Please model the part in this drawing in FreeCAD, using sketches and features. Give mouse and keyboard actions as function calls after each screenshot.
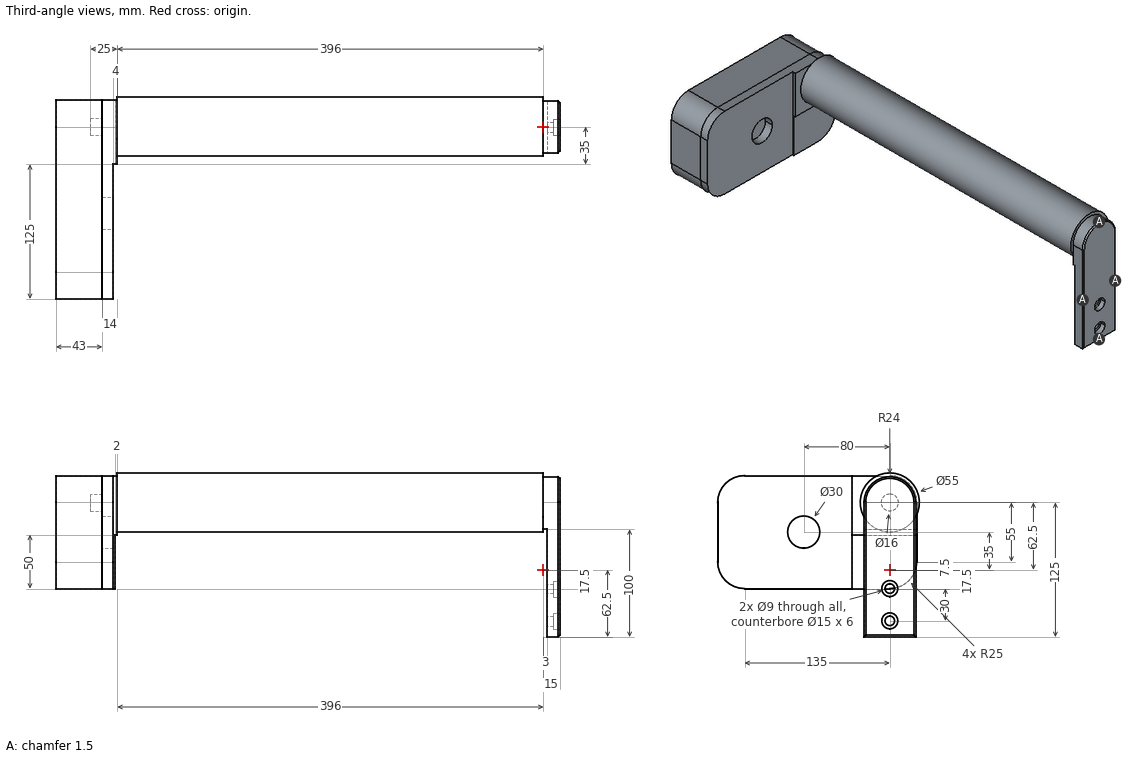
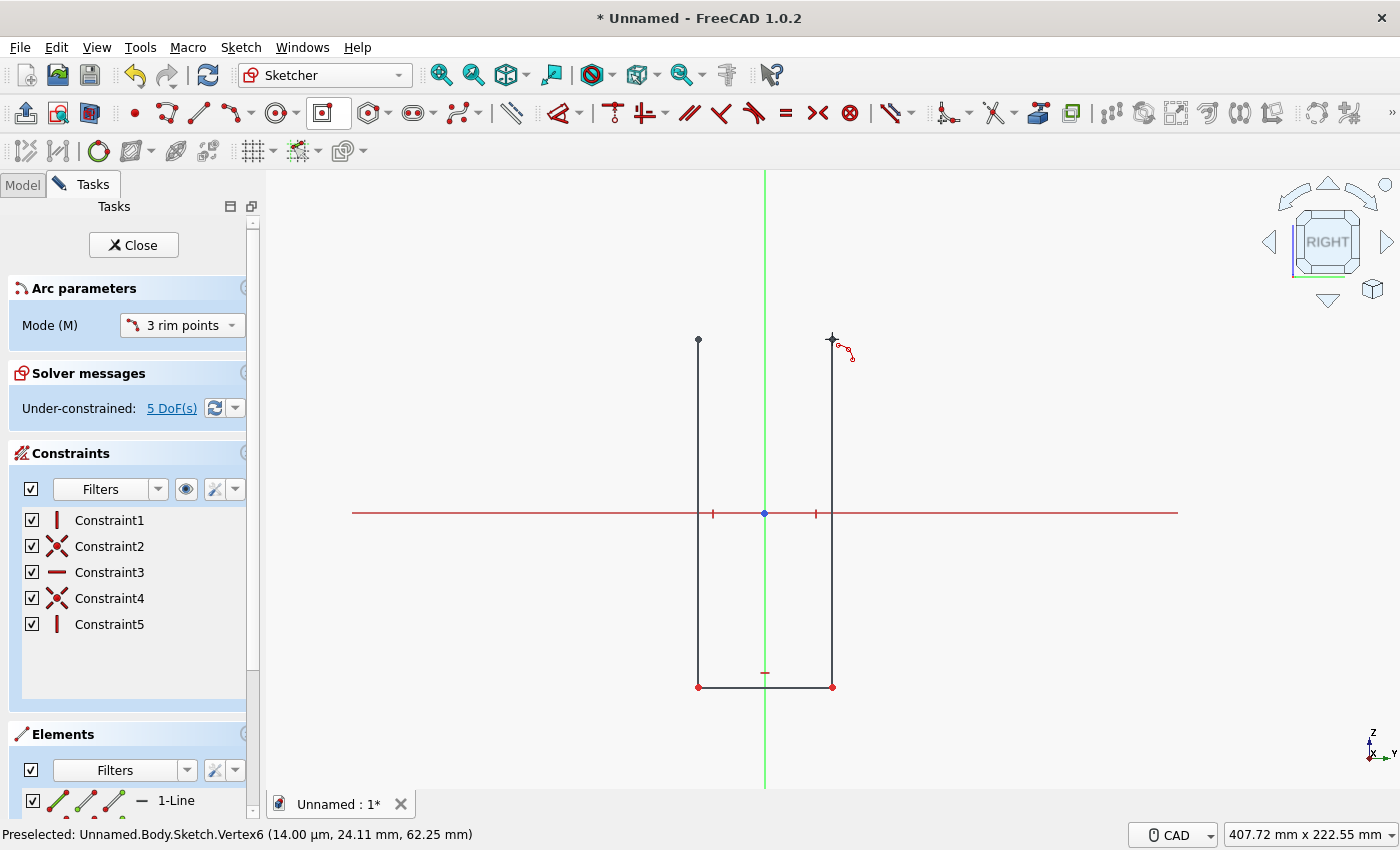
click(832, 340)
click(698, 340)
click(786, 276)
key(Escape)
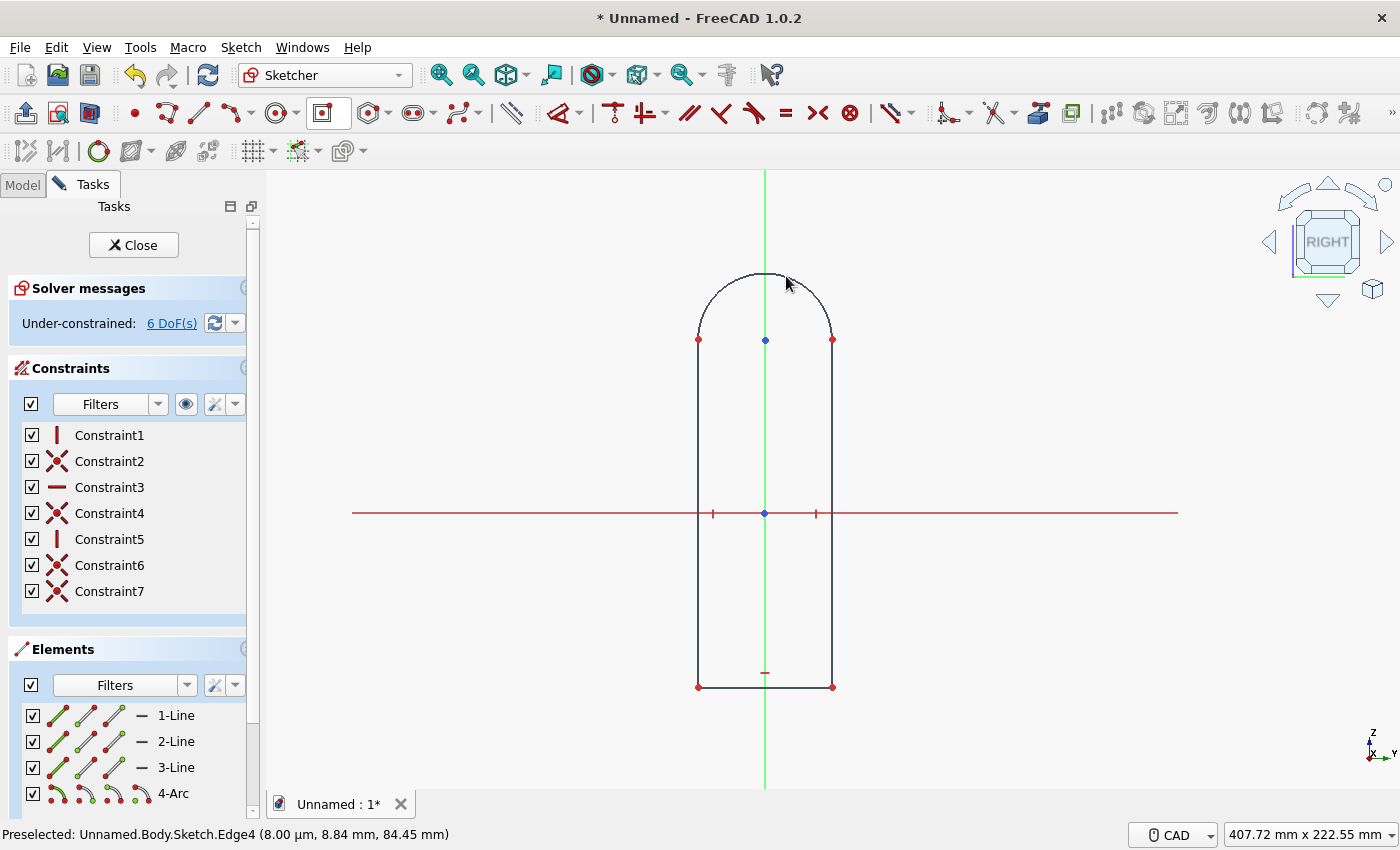
click(698, 444)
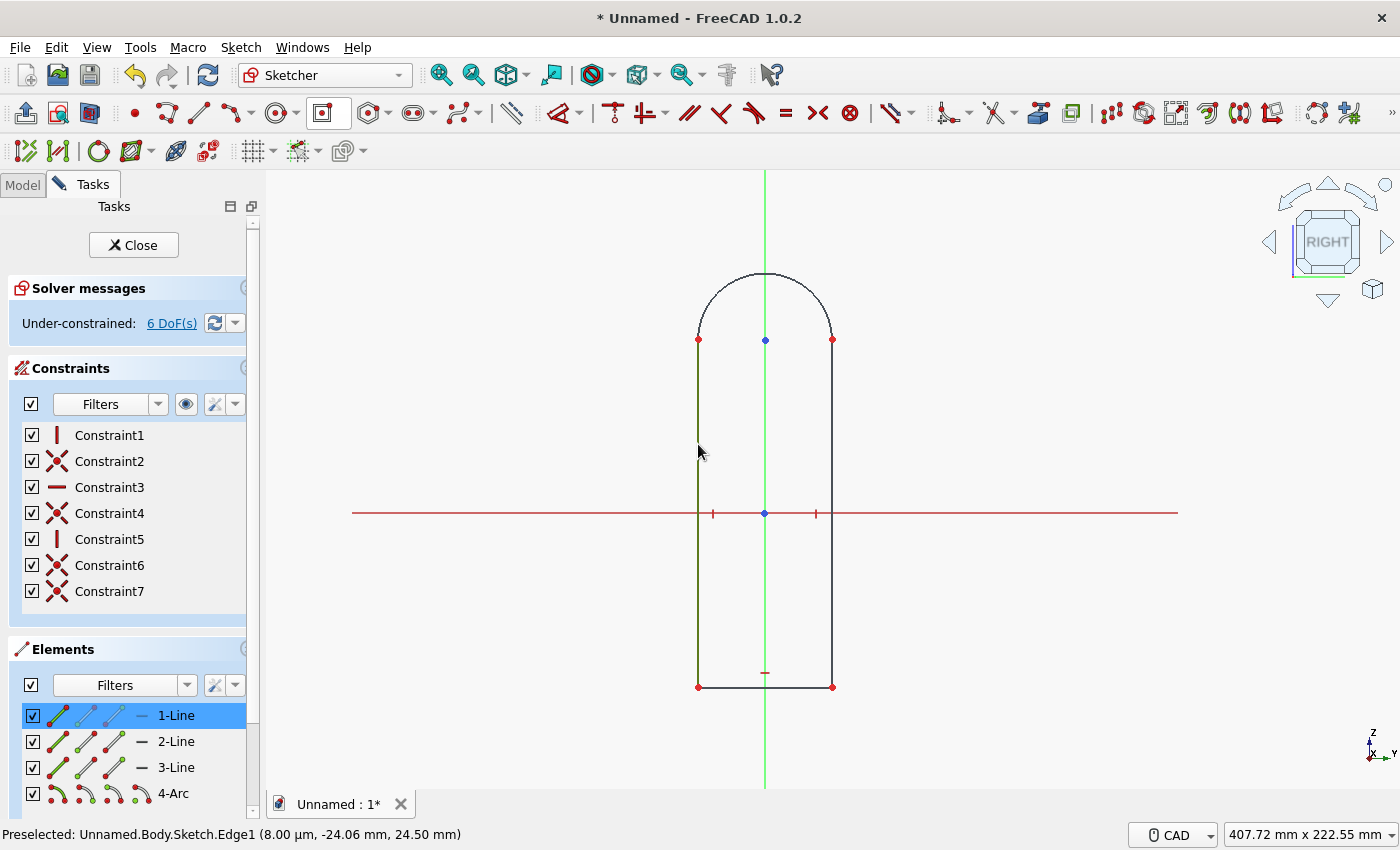
click(804, 286)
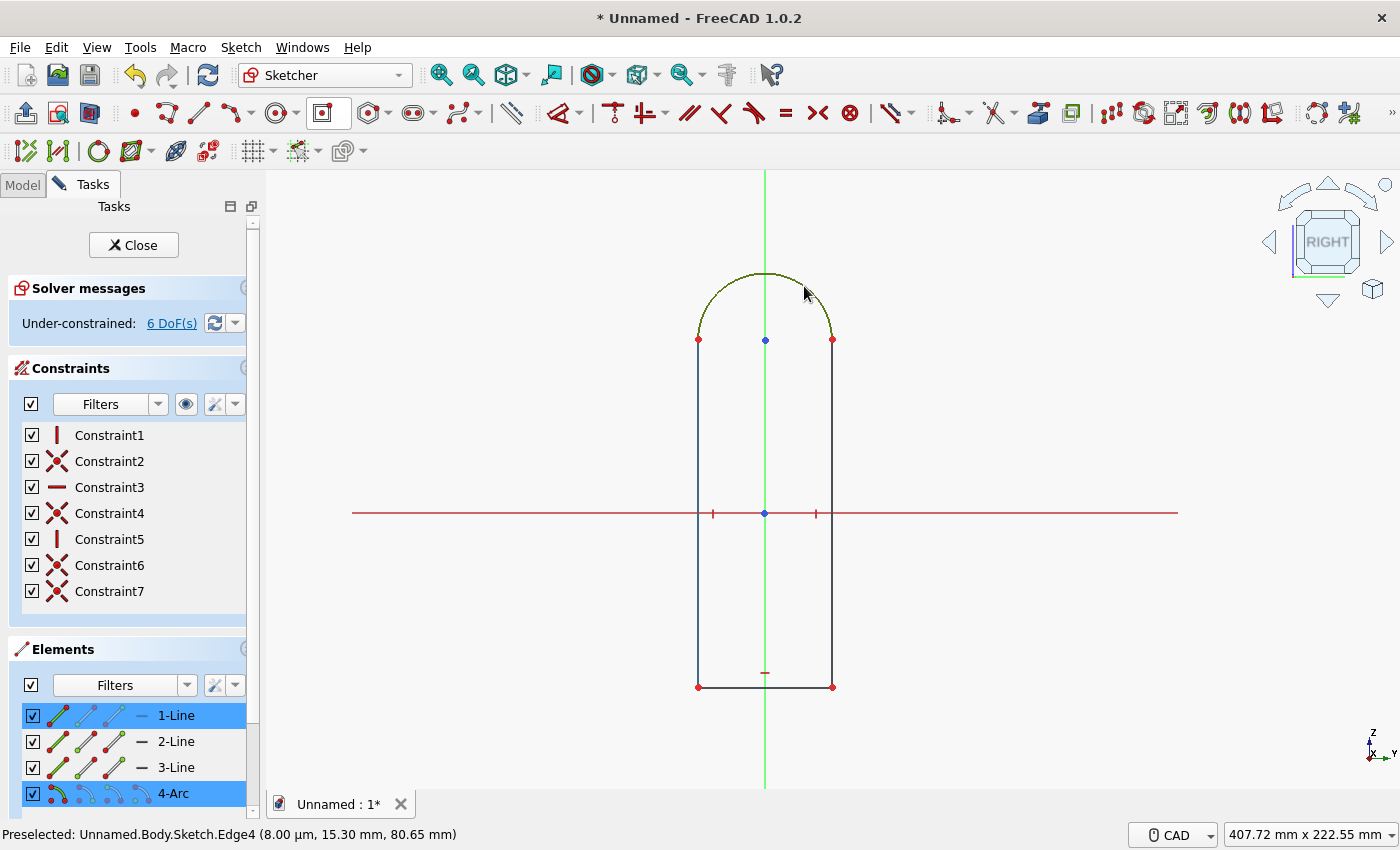
click(754, 114)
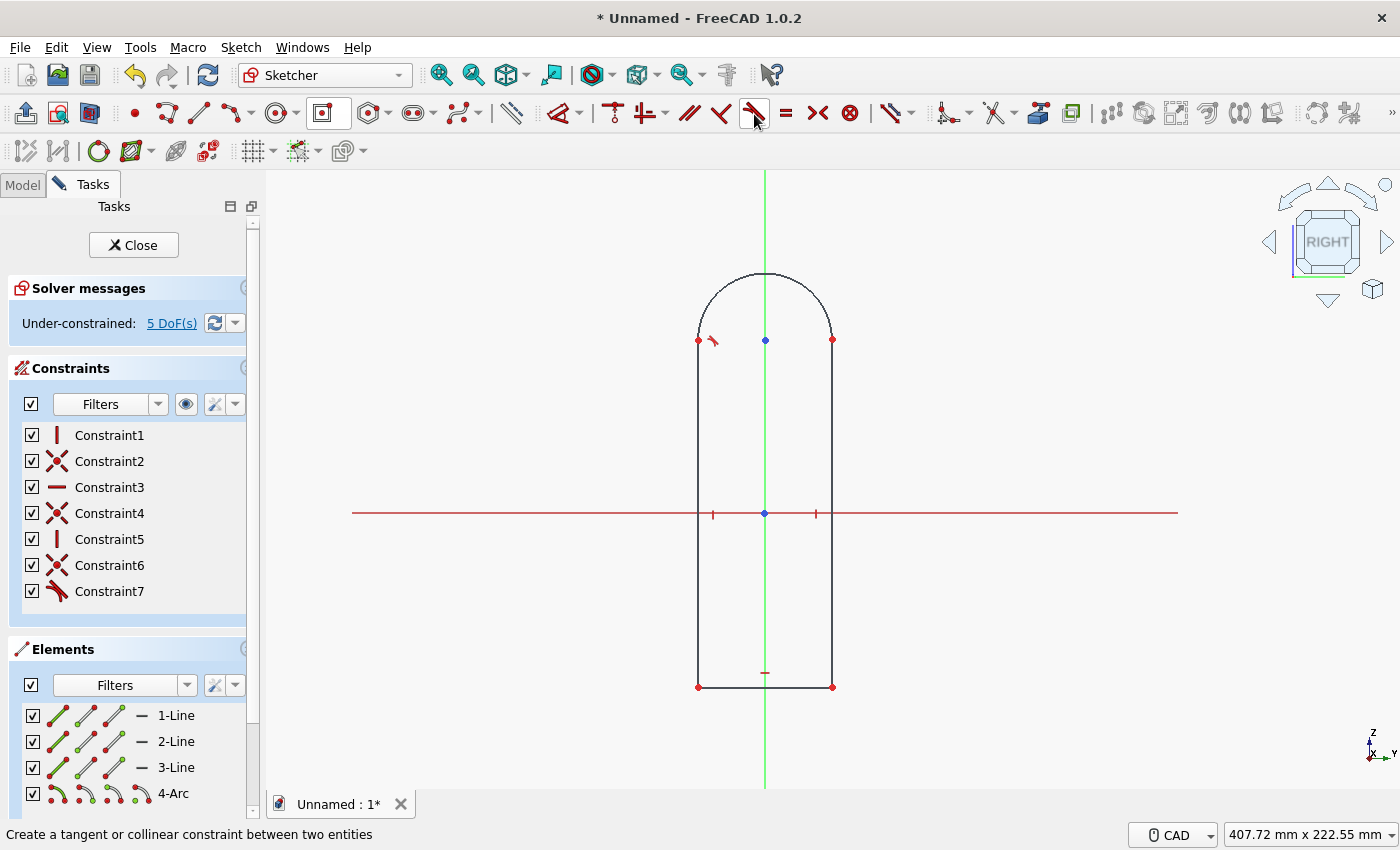
click(832, 584)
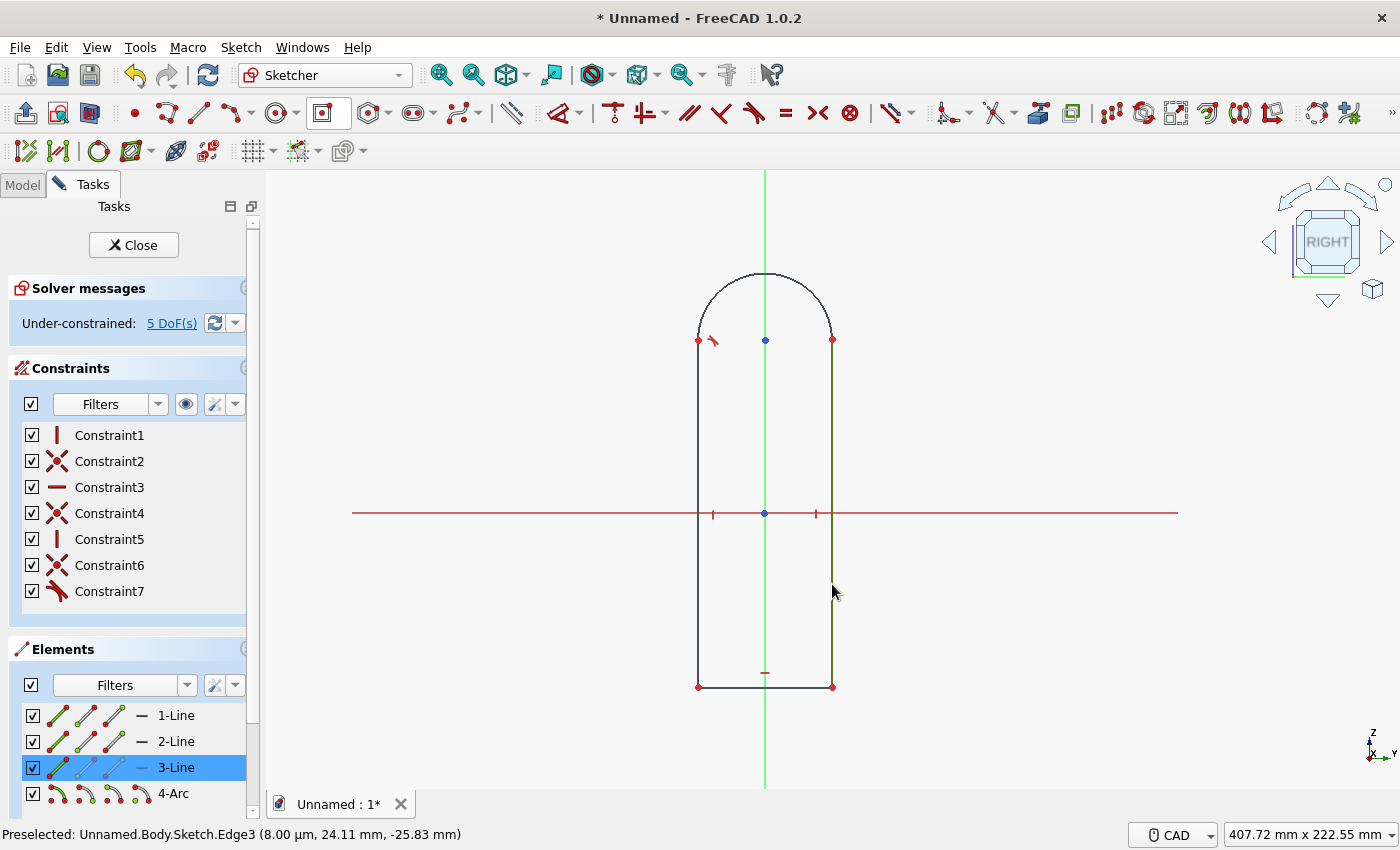
click(804, 286)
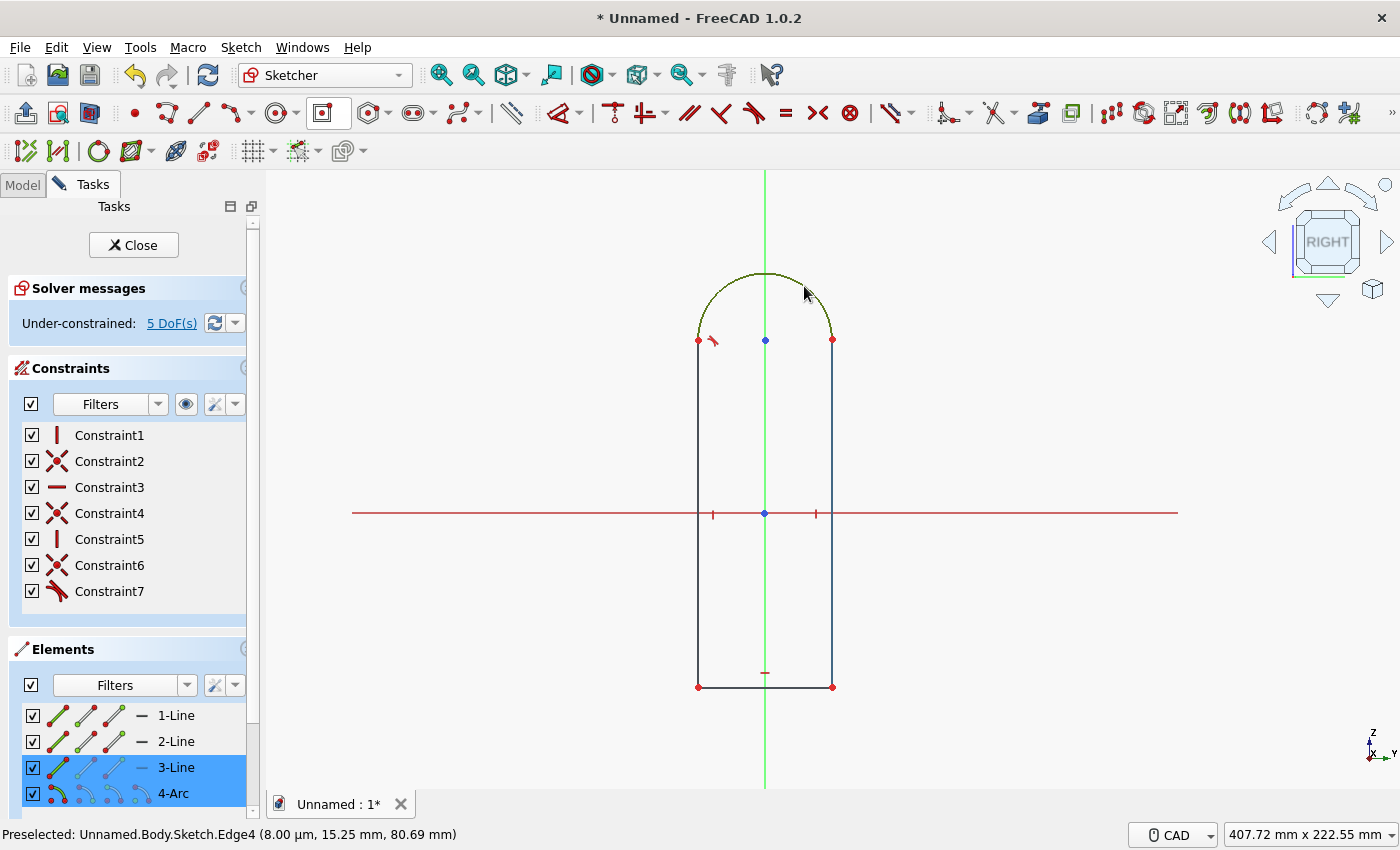
key(t)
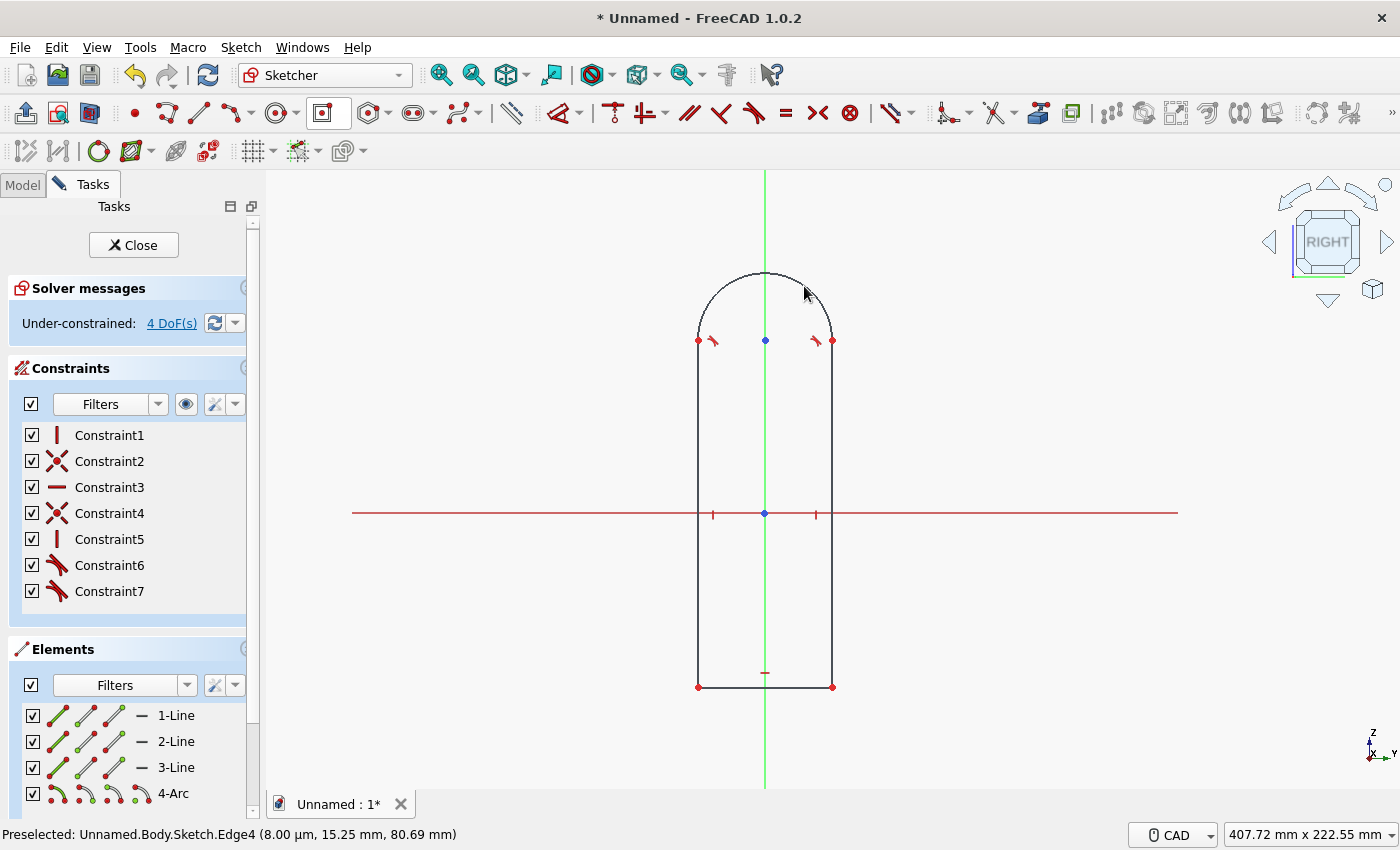
click(765, 340)